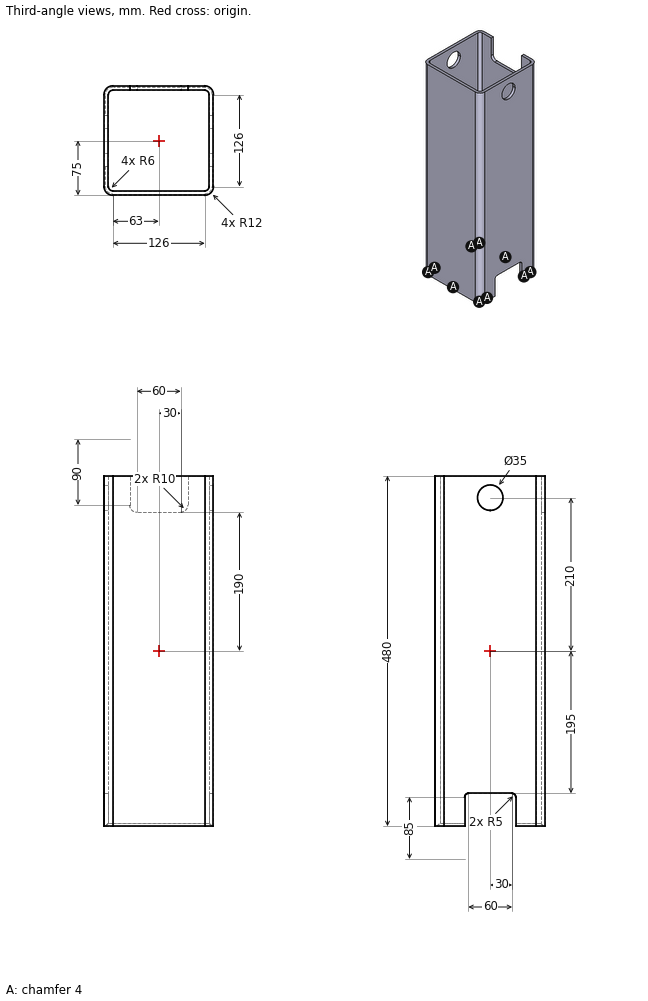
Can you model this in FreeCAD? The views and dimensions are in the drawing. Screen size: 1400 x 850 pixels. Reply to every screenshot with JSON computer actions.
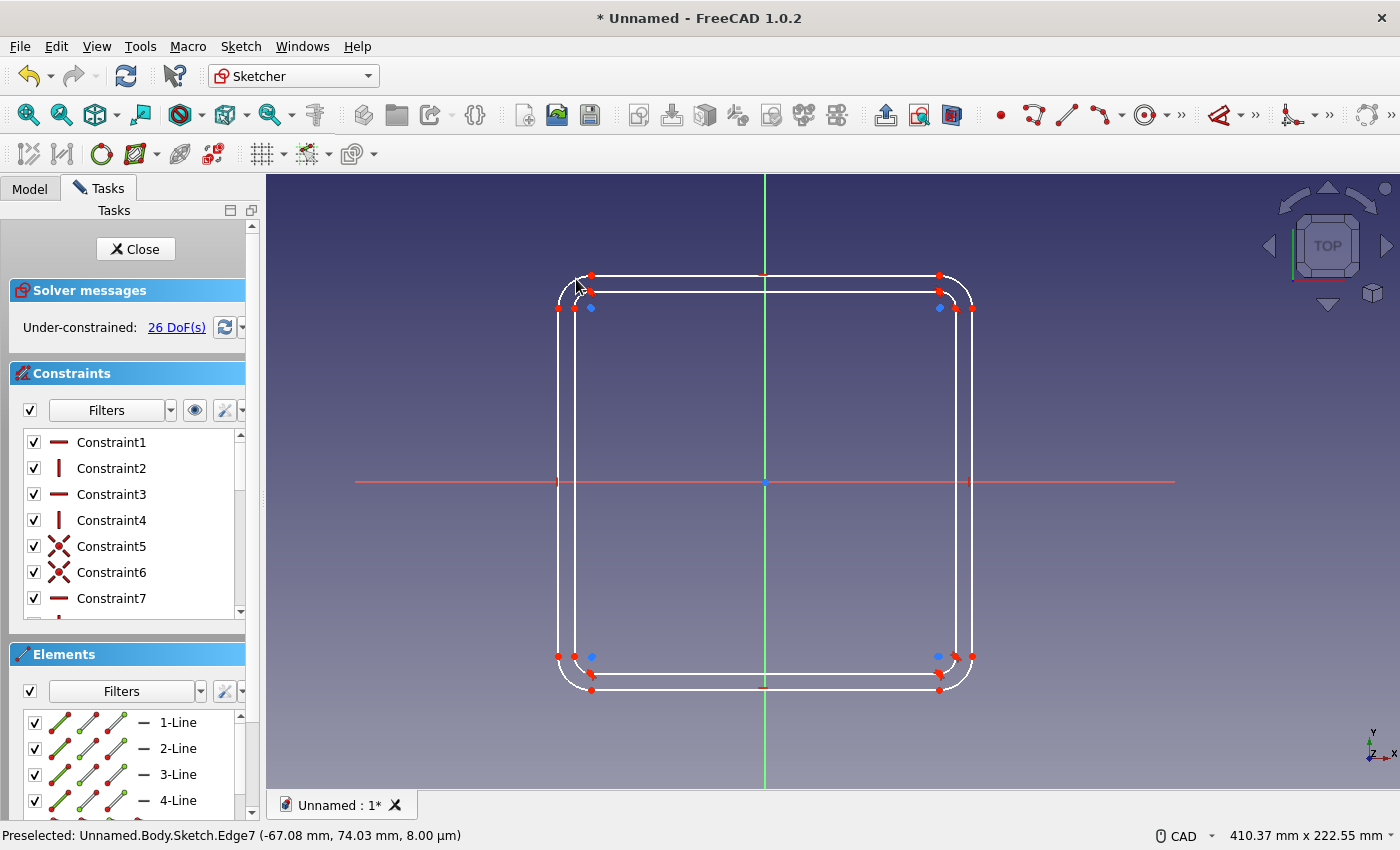
{"action": "left_click", "coordinate": [558, 413]}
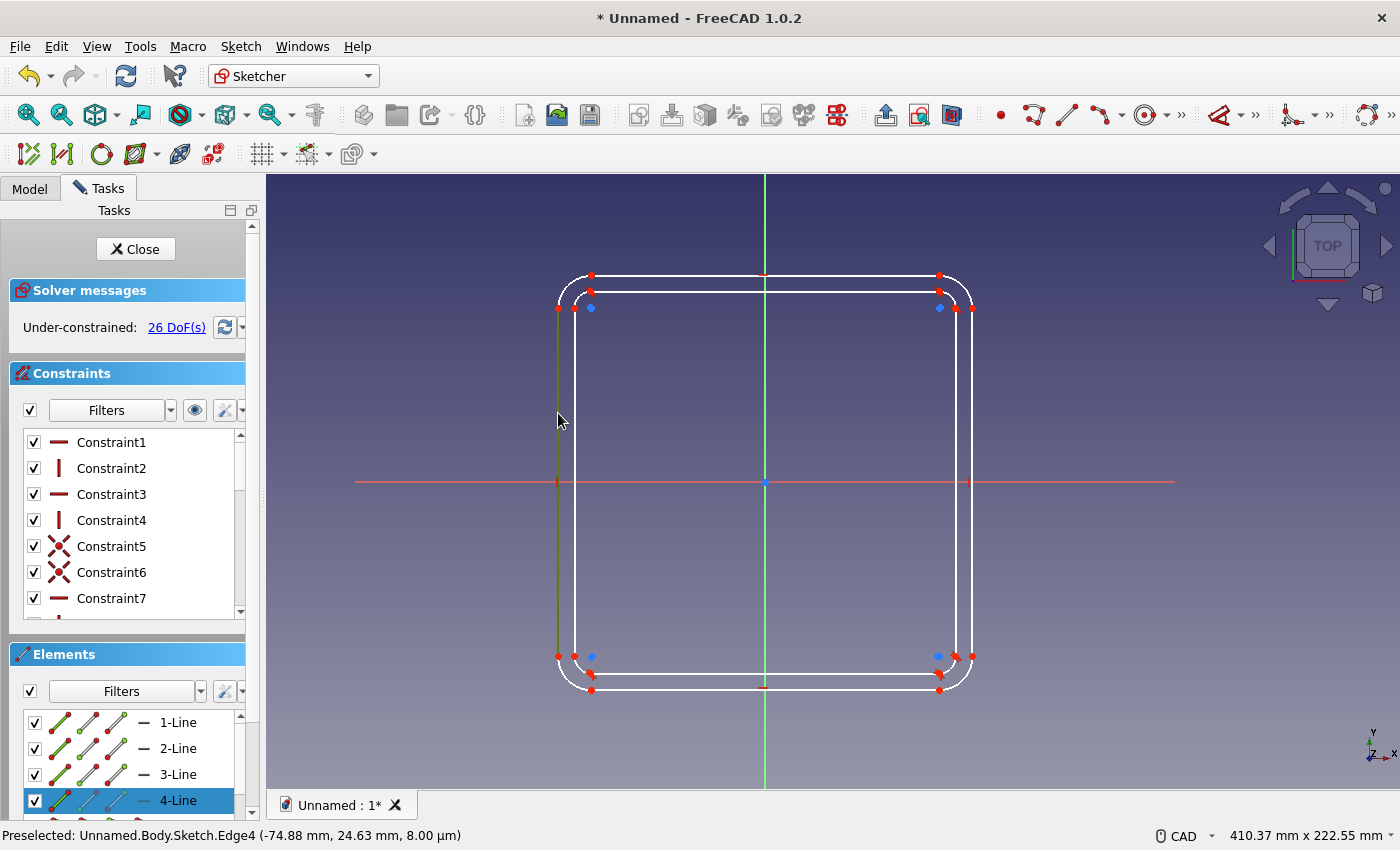
{"action": "left_click", "coordinate": [576, 280]}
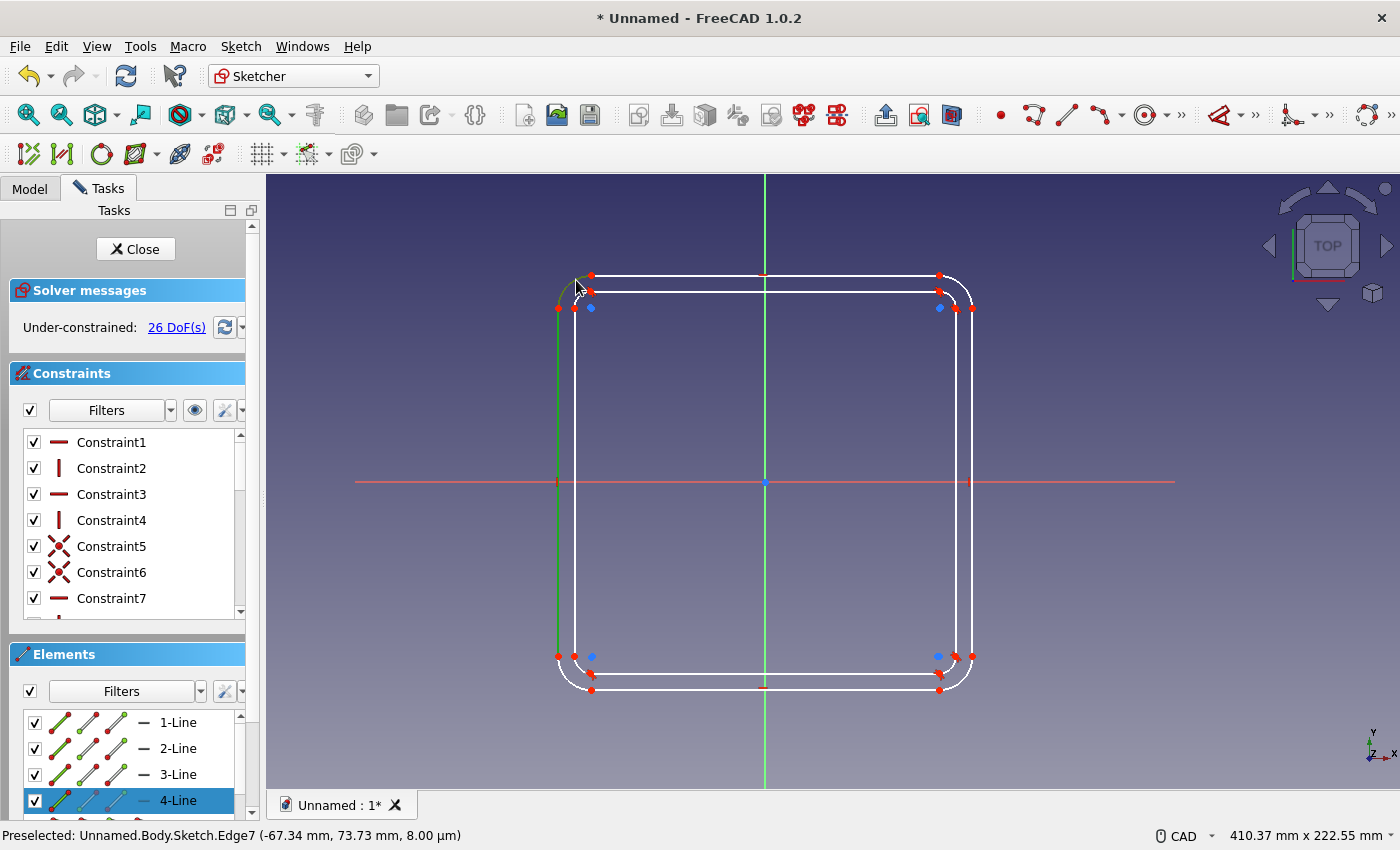
{"action": "key", "text": "t"}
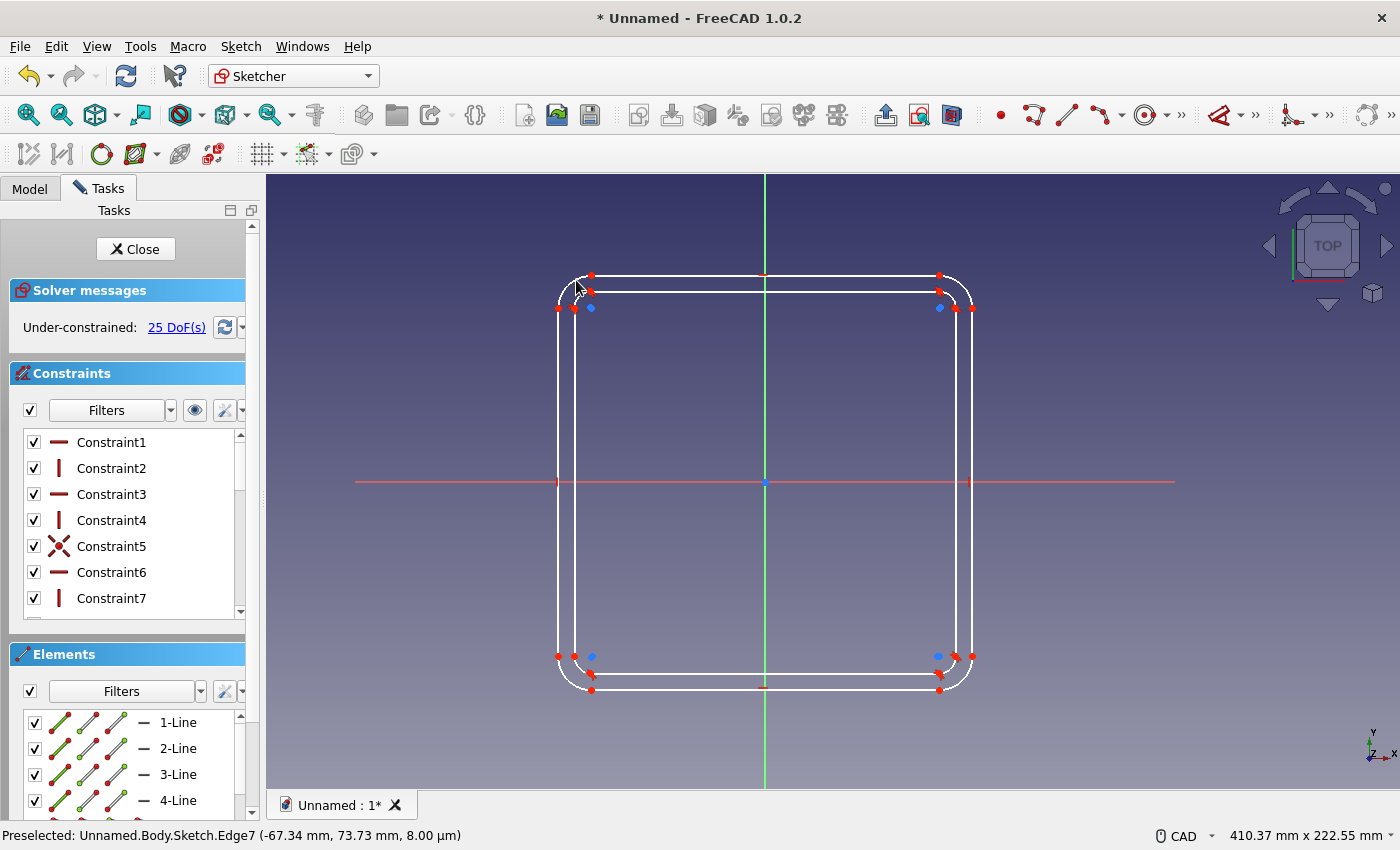
{"action": "left_click", "coordinate": [558, 413]}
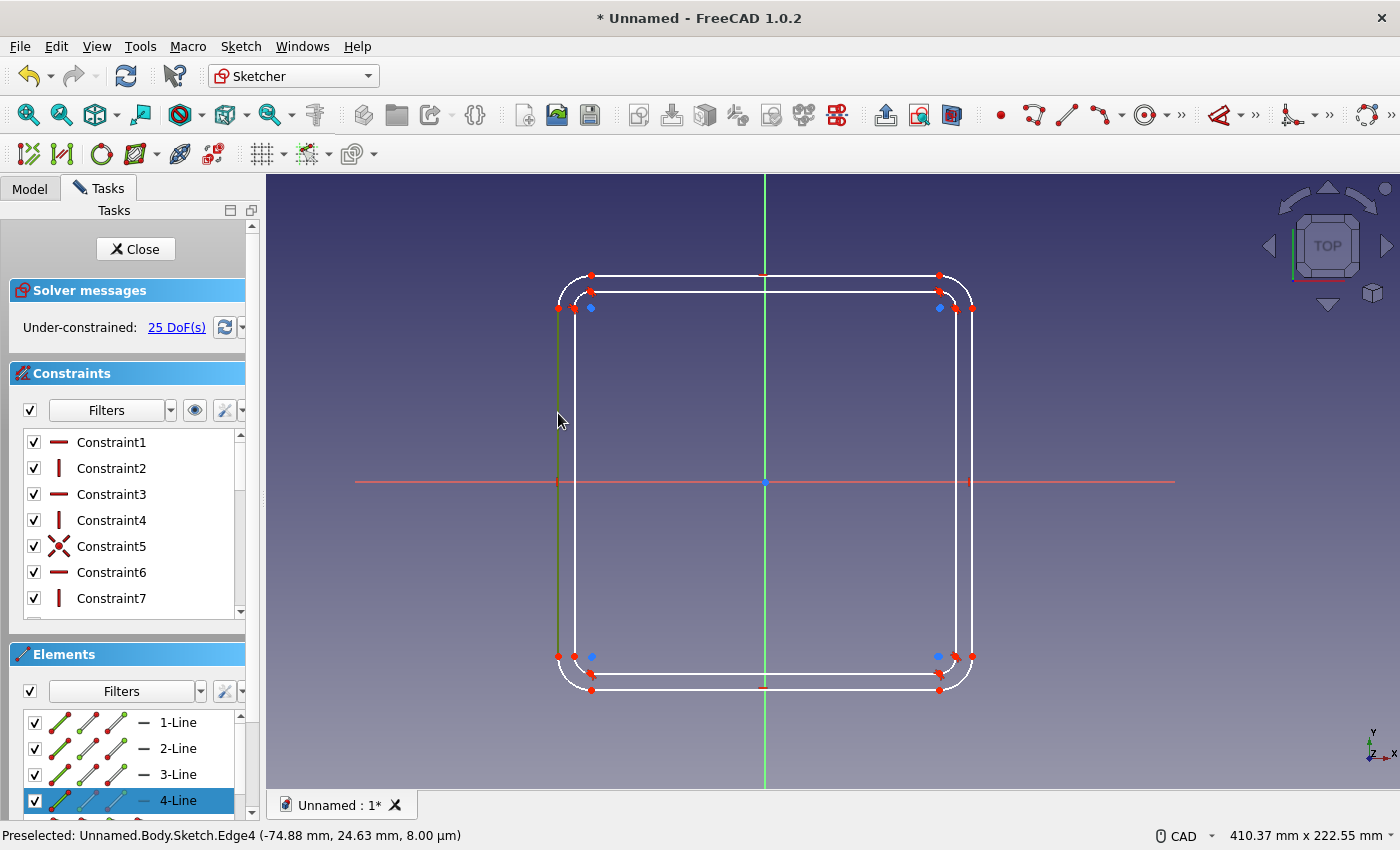
{"action": "left_click", "coordinate": [562, 672]}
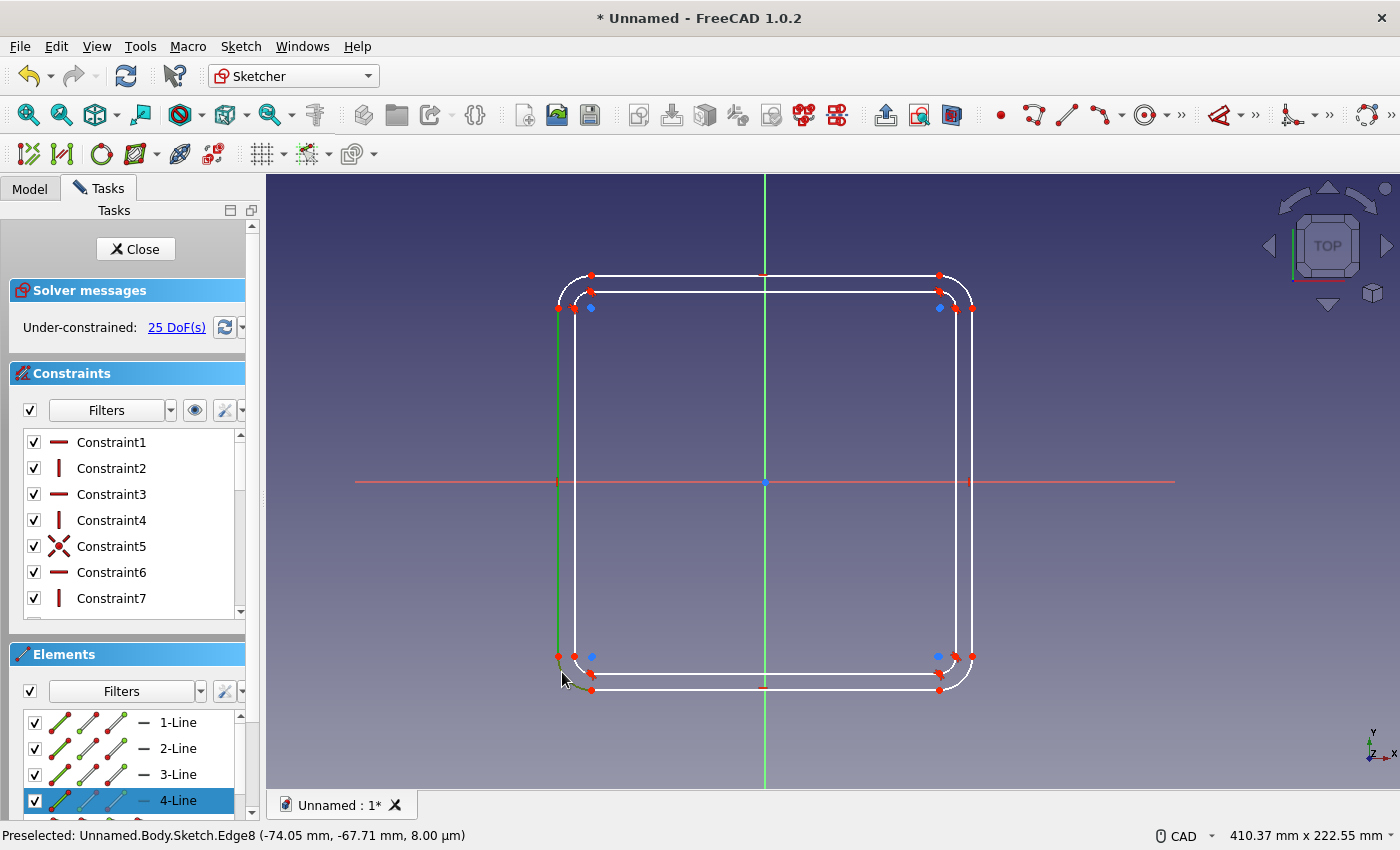
{"action": "key", "text": "t"}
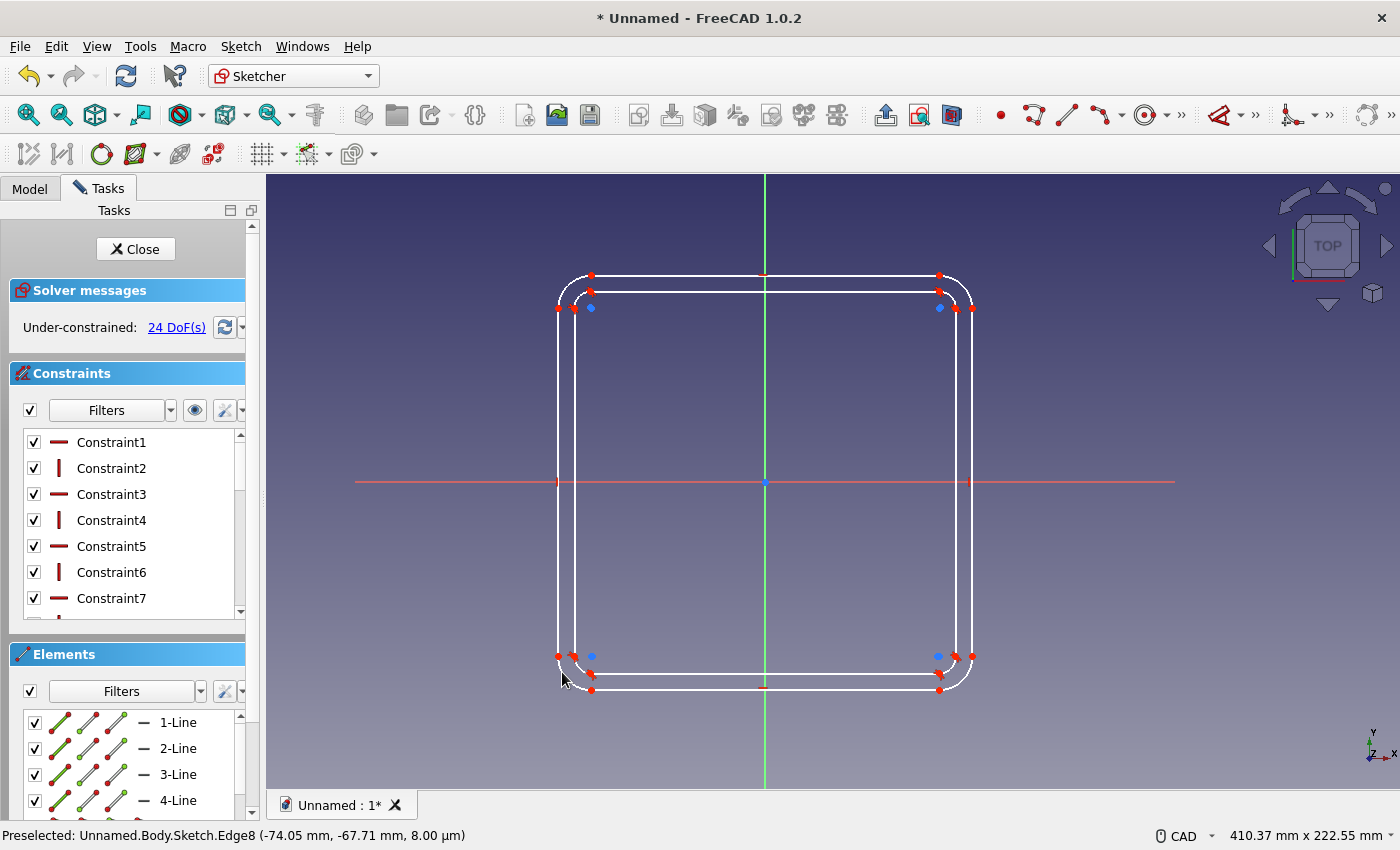
{"action": "left_click", "coordinate": [835, 674]}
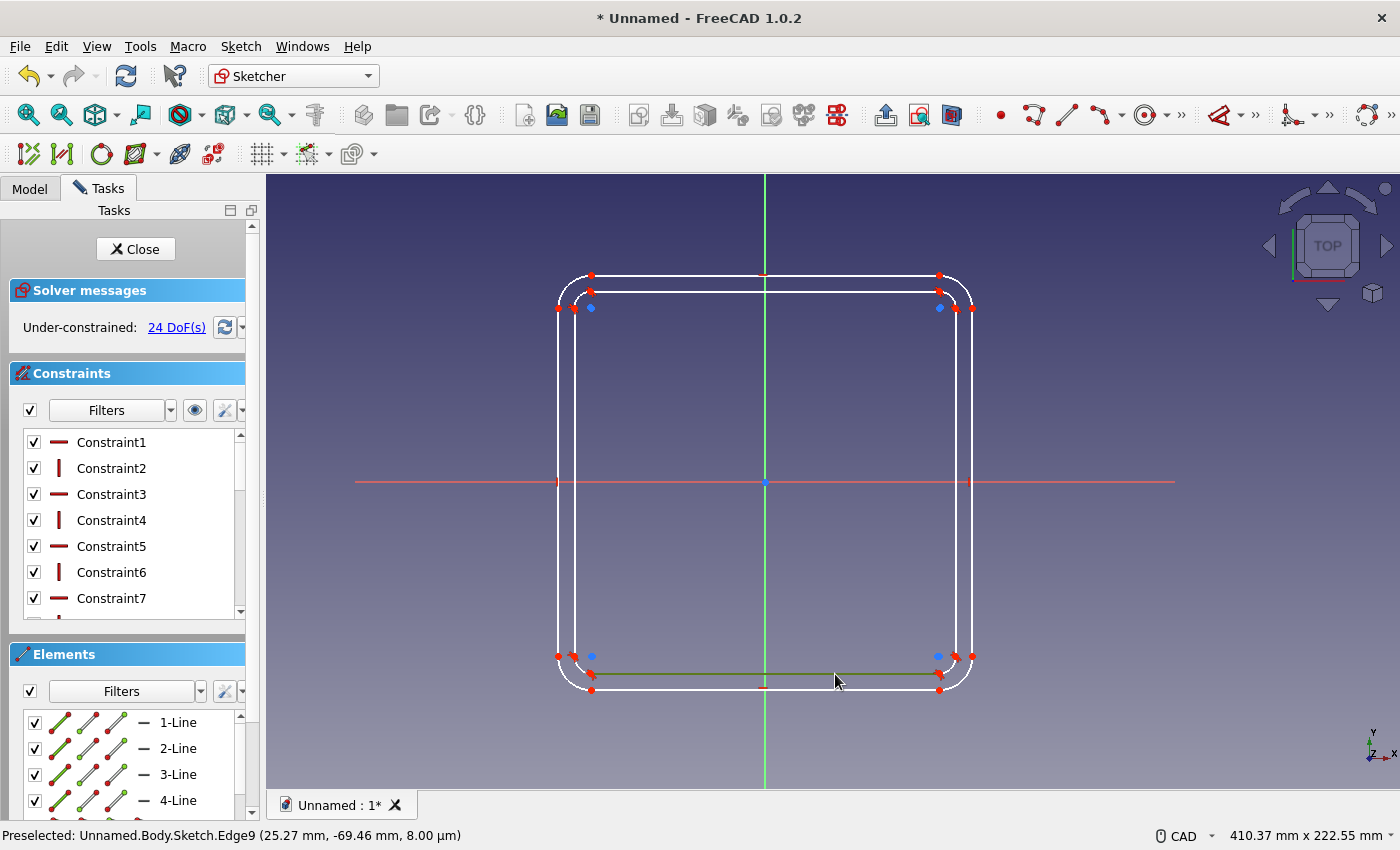
{"action": "left_click", "coordinate": [580, 669]}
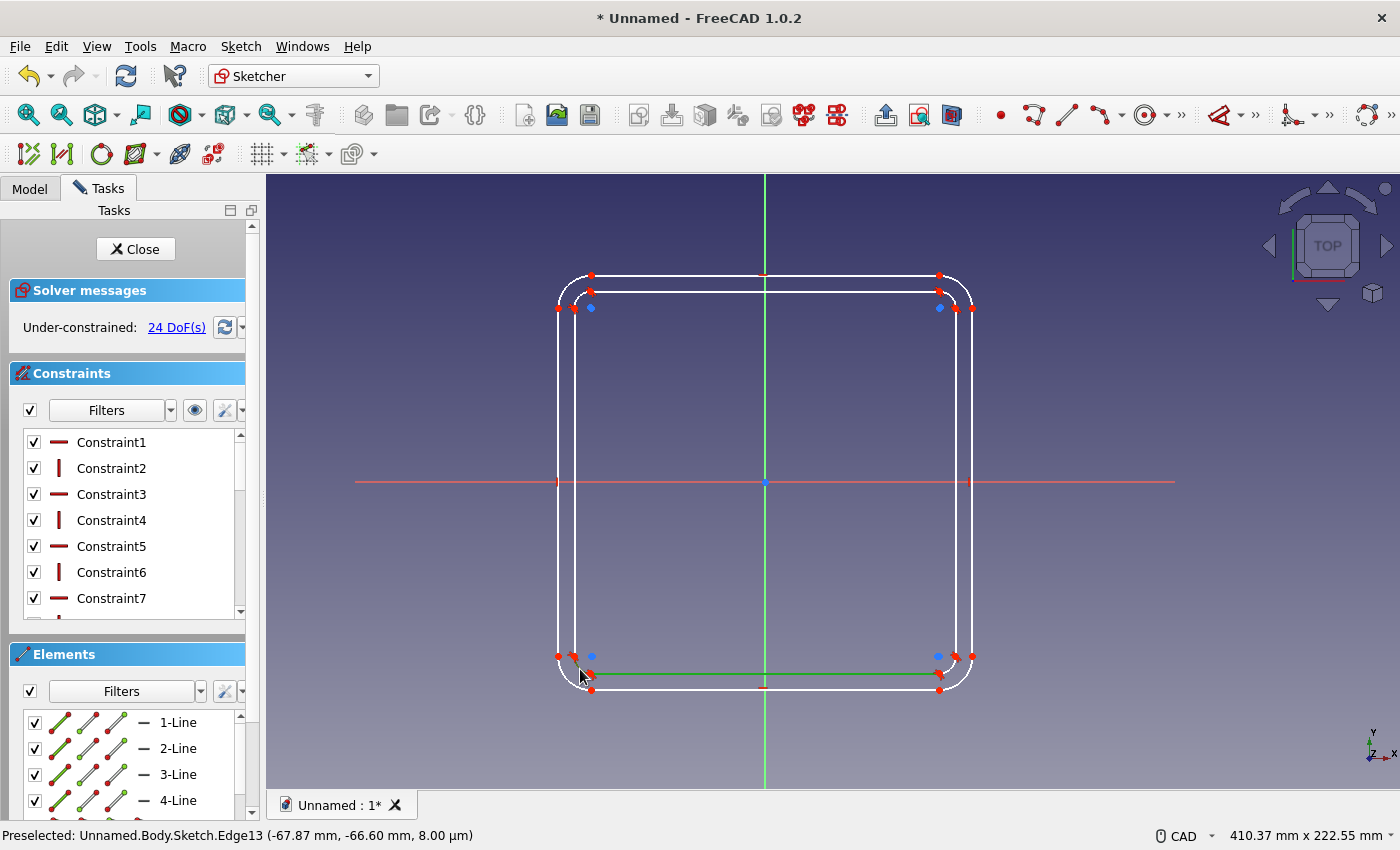
{"action": "key", "text": "t"}